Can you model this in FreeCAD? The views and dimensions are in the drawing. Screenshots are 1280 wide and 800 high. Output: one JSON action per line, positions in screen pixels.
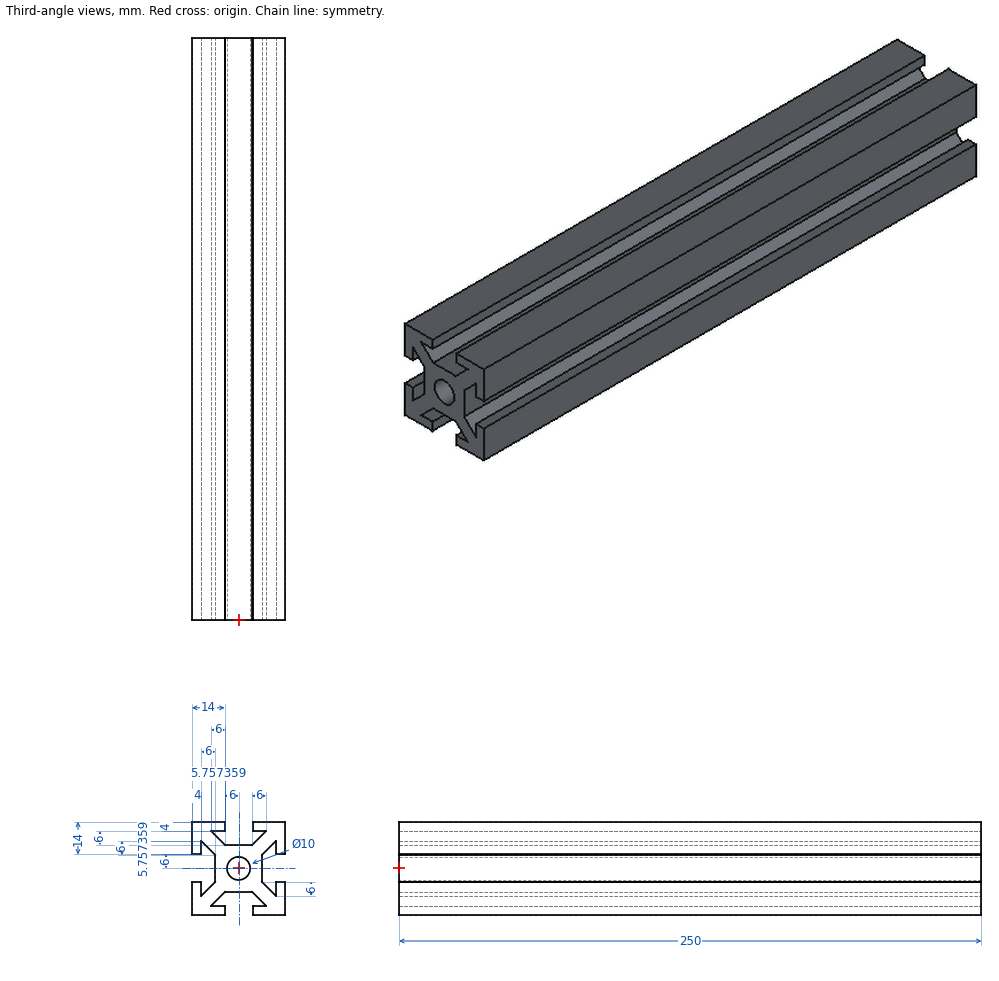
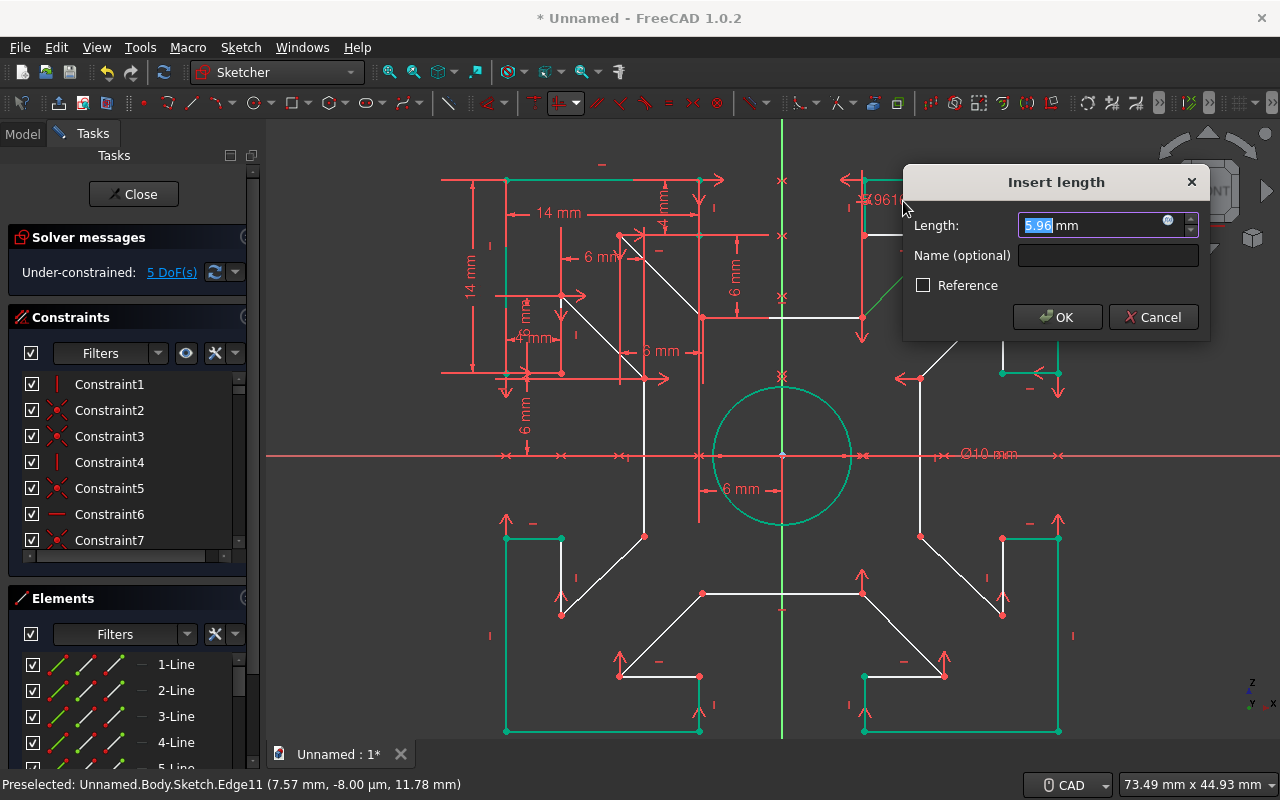
{"action": "type", "text": "6"}
{"action": "key", "text": "Return"}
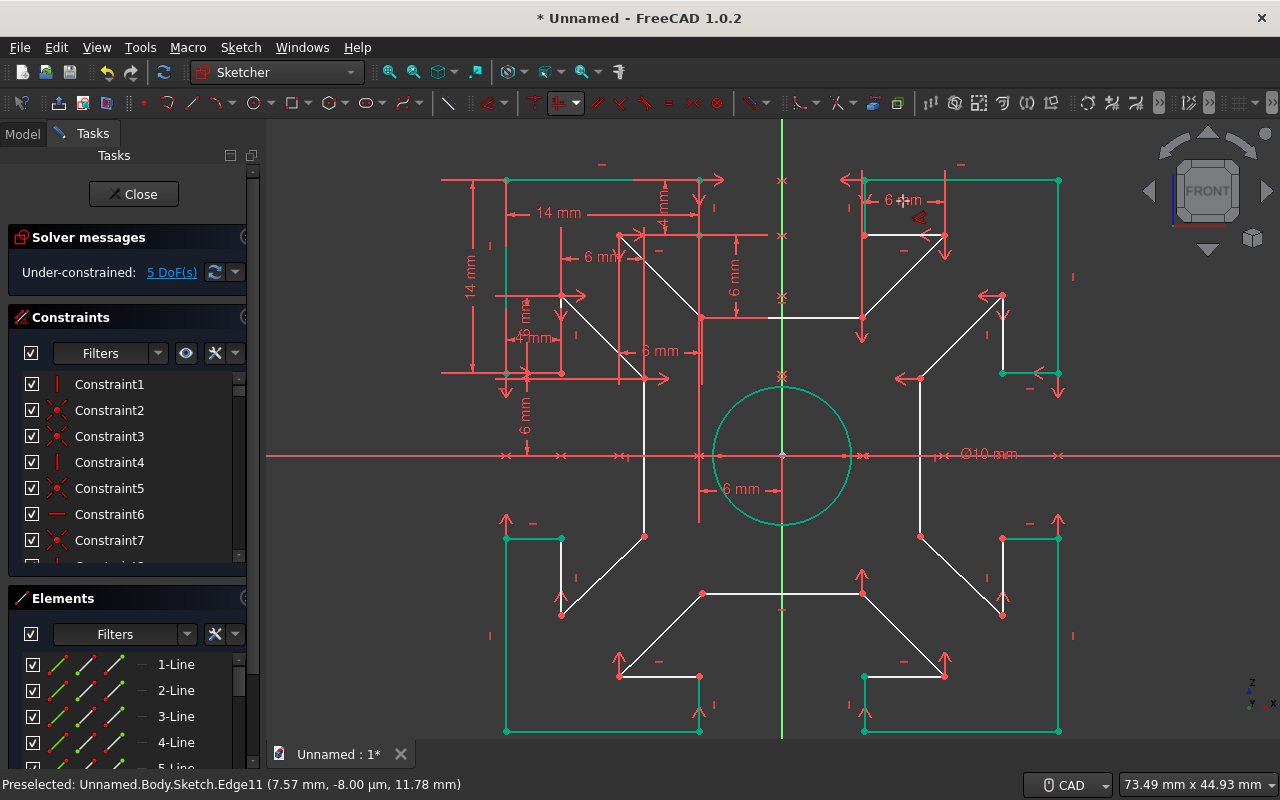
{"action": "left_click", "coordinate": [945, 561]}
{"action": "left_click", "coordinate": [1037, 576]}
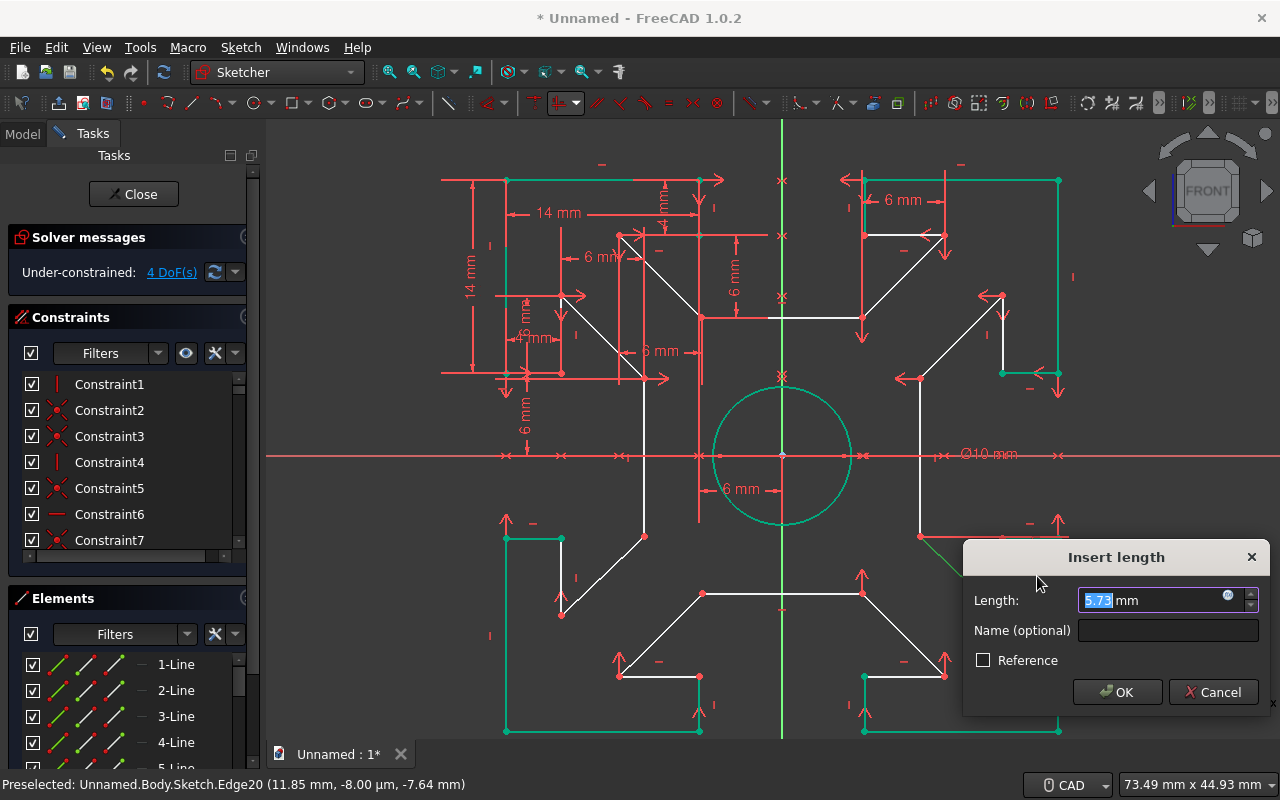
{"action": "type", "text": "6"}
{"action": "key", "text": "Return"}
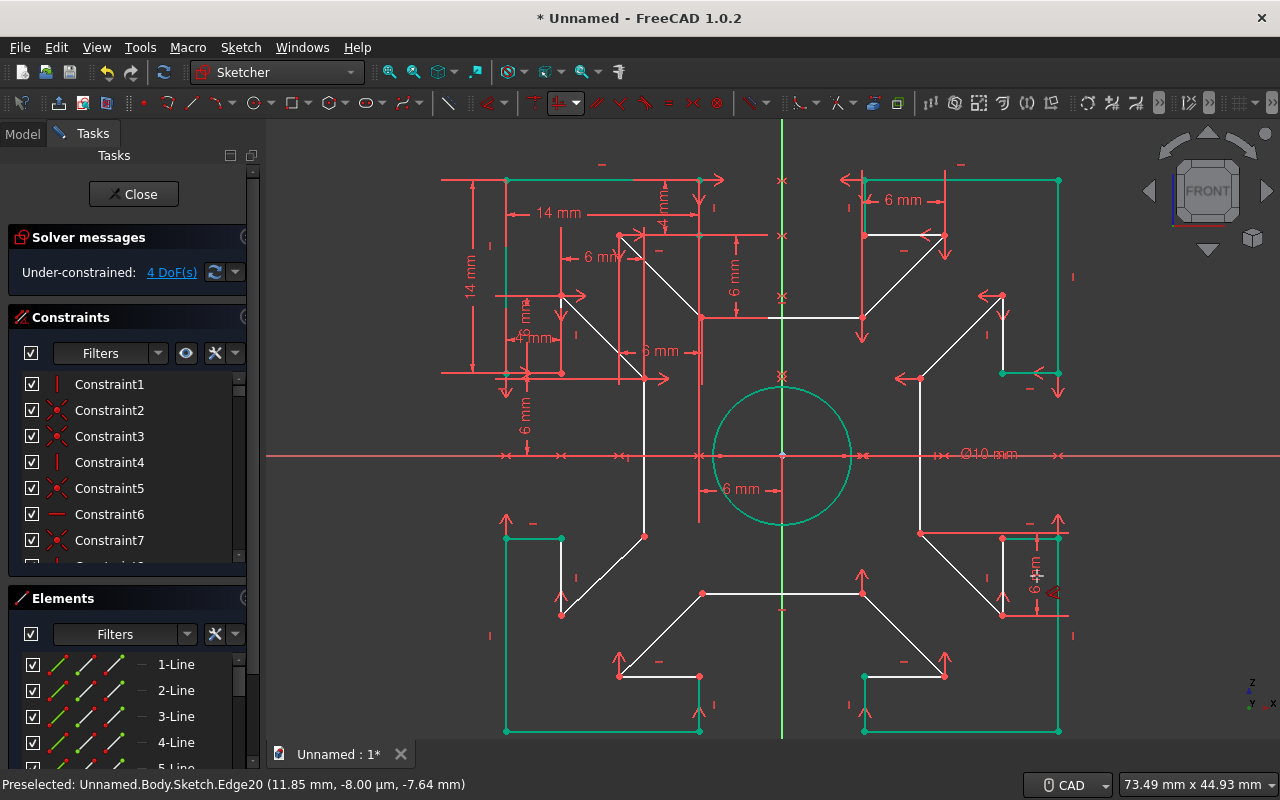
{"action": "left_click", "coordinate": [678, 619]}
{"action": "left_click", "coordinate": [661, 711]}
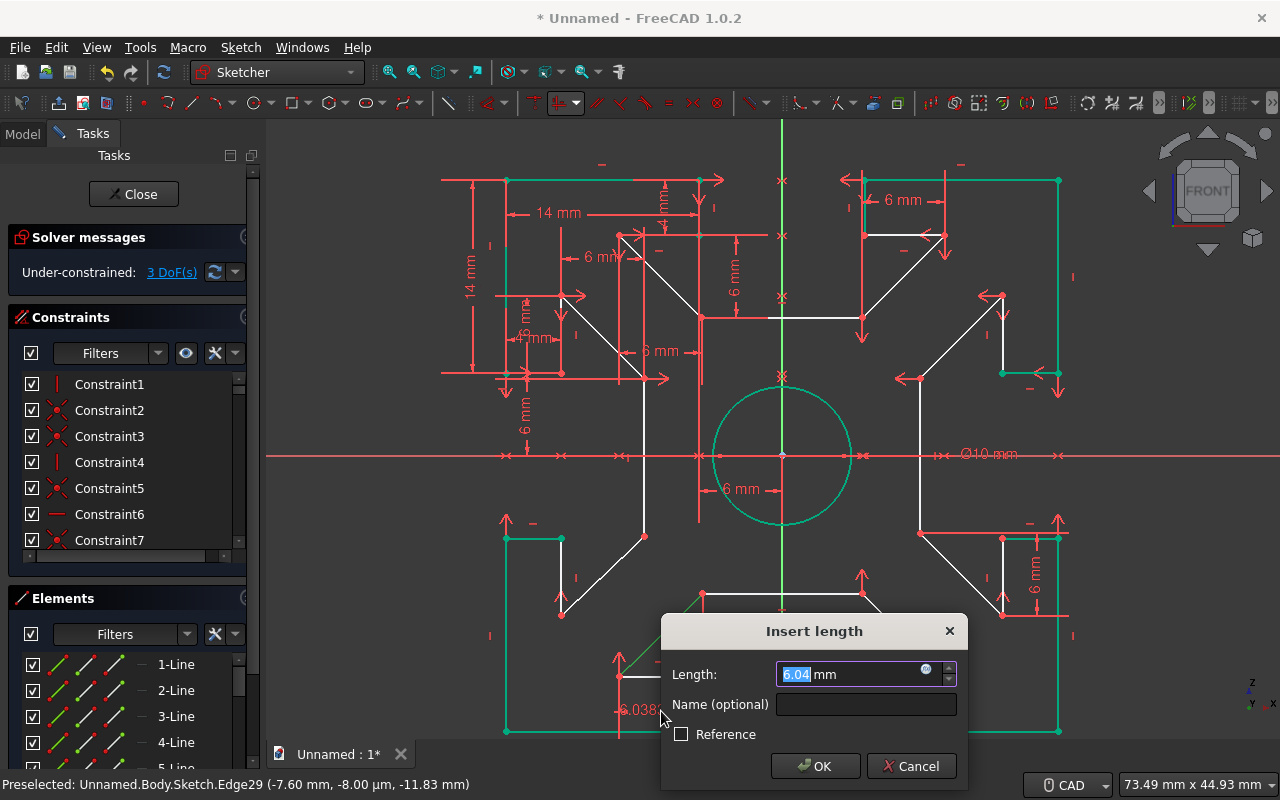
{"action": "type", "text": "6"}
{"action": "key", "text": "Return"}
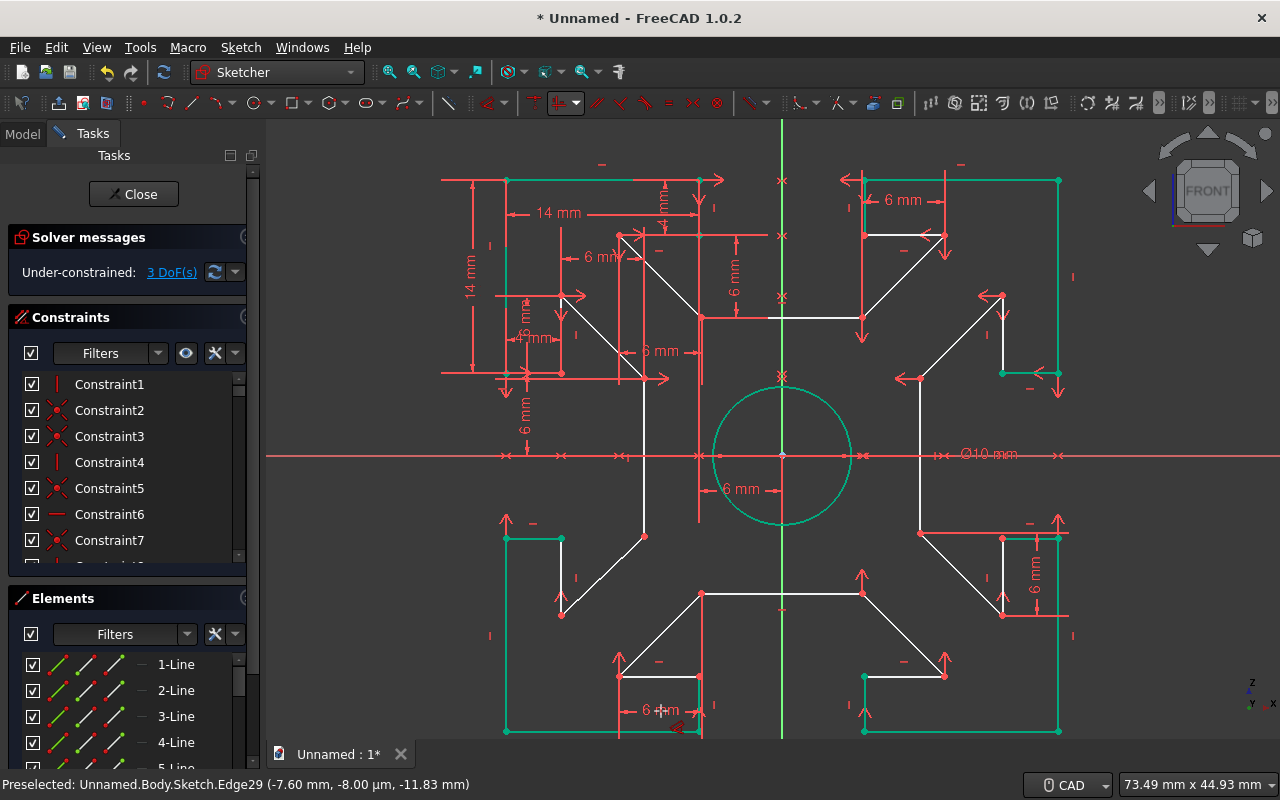
{"action": "left_click", "coordinate": [586, 592]}
{"action": "left_click", "coordinate": [527, 576]}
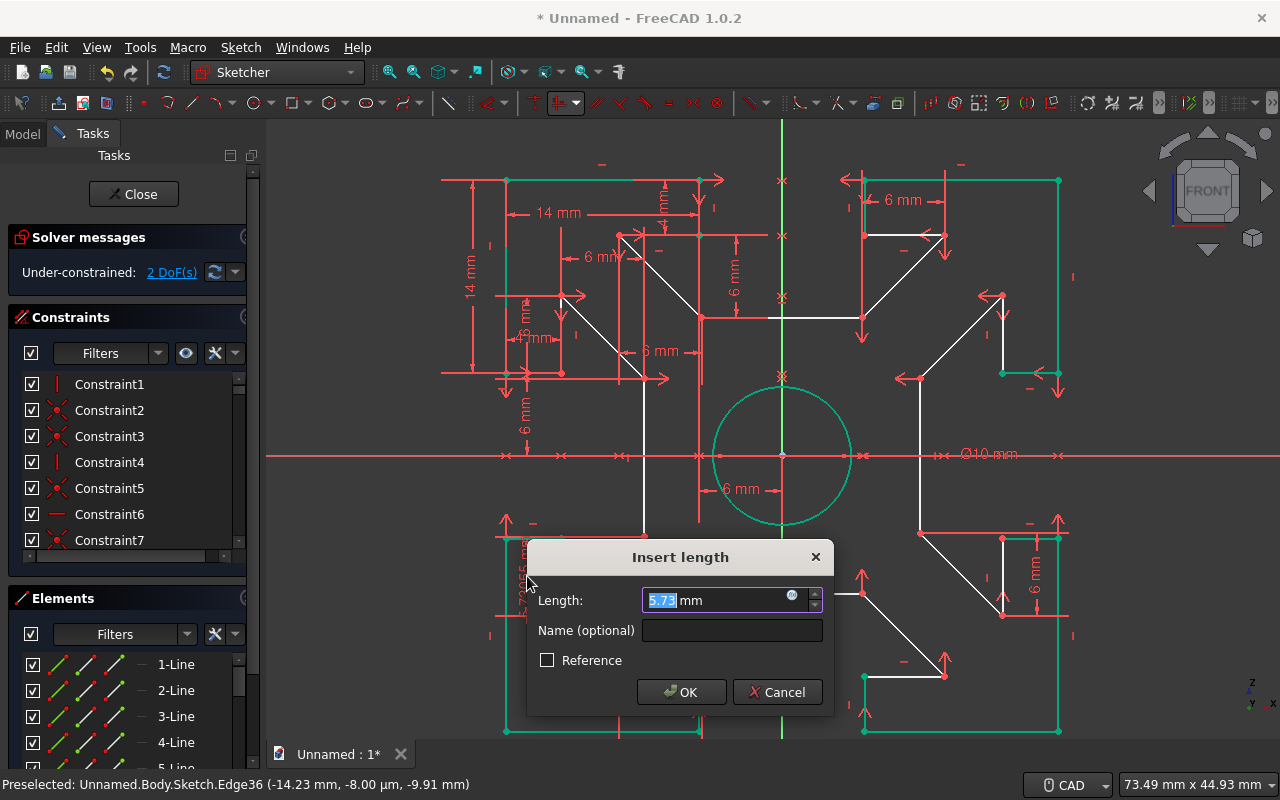
{"action": "type", "text": "6"}
{"action": "key", "text": "Return"}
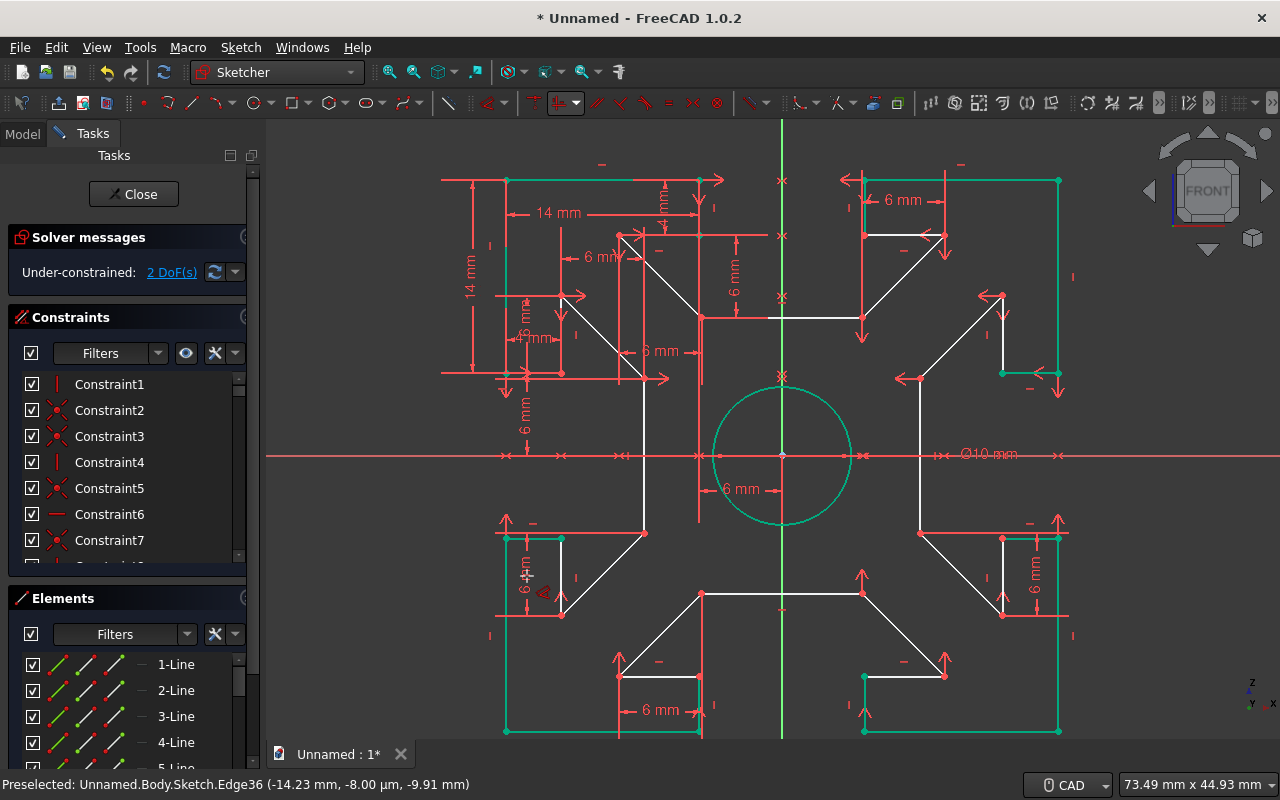
{"action": "left_click", "coordinate": [561, 319]}
{"action": "left_click", "coordinate": [619, 317]}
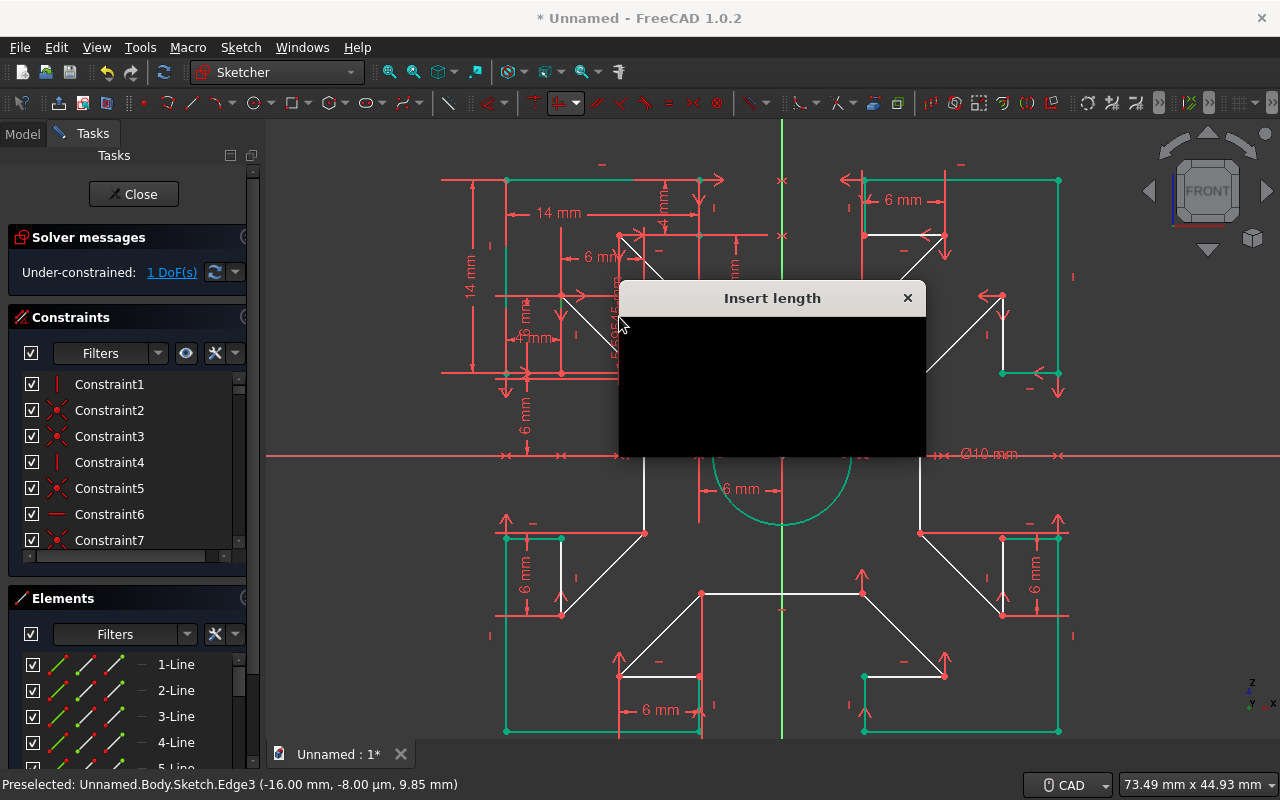
{"action": "type", "text": "5.757359"}
{"action": "key", "text": "Return"}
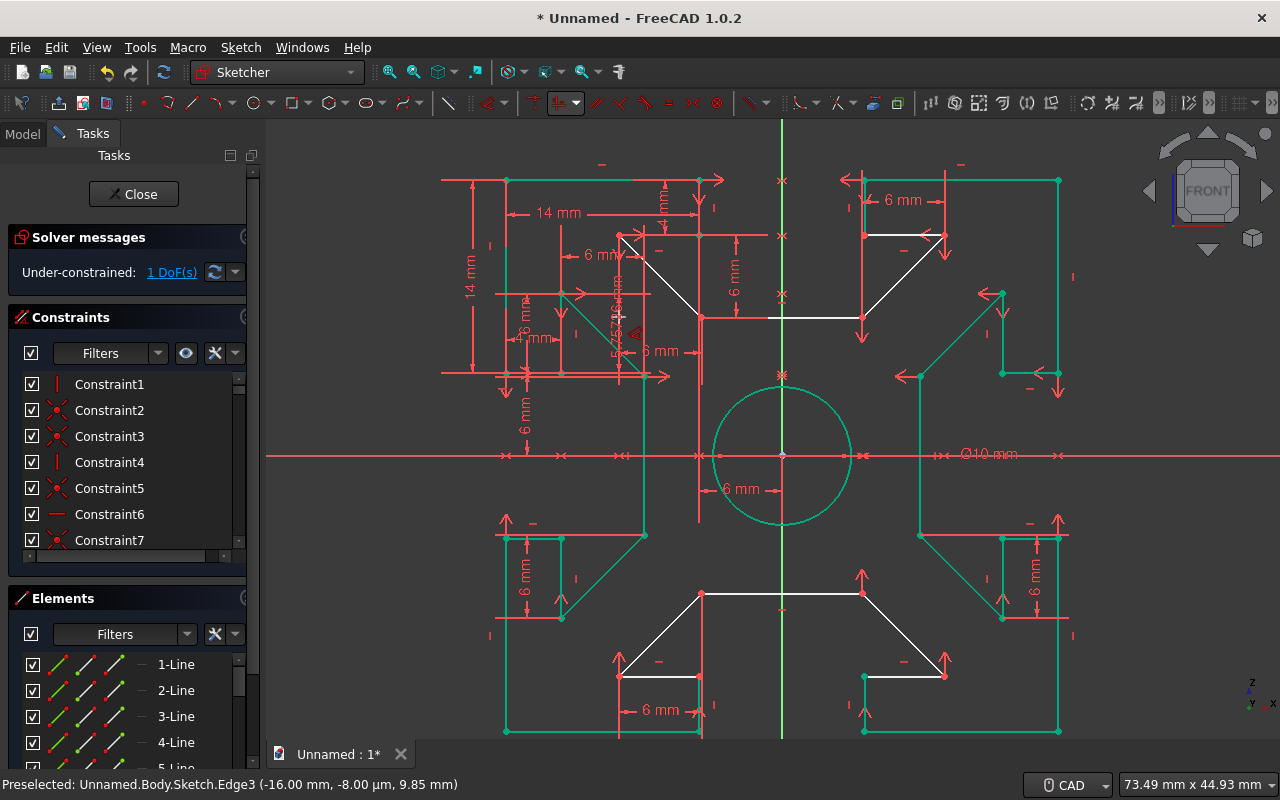
{"action": "left_click", "coordinate": [675, 235]}
{"action": "left_click", "coordinate": [641, 293]}